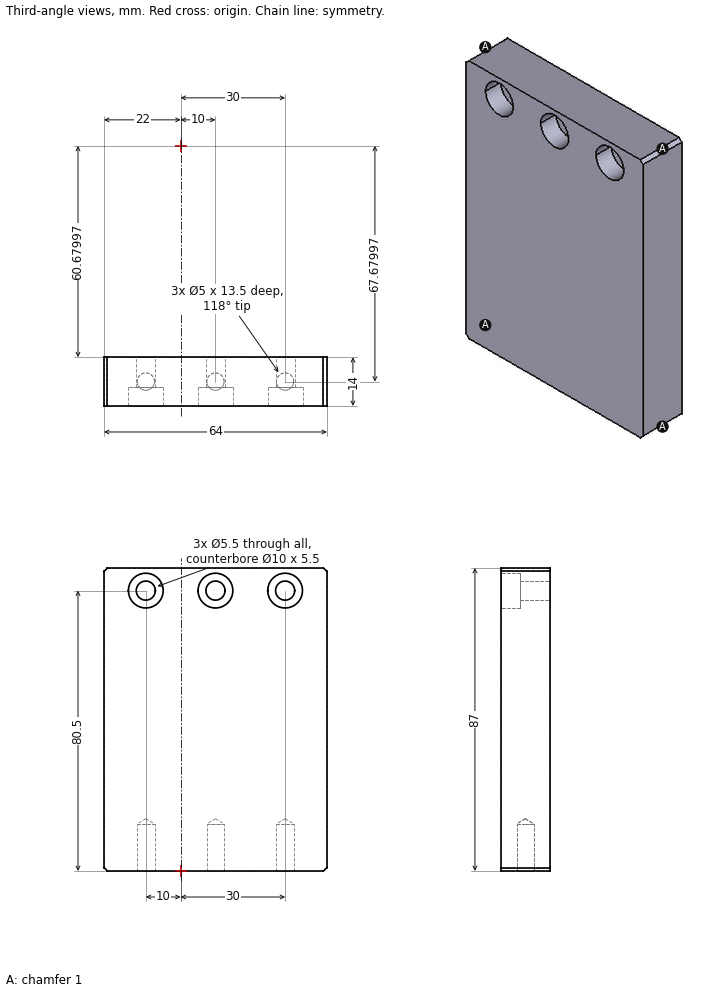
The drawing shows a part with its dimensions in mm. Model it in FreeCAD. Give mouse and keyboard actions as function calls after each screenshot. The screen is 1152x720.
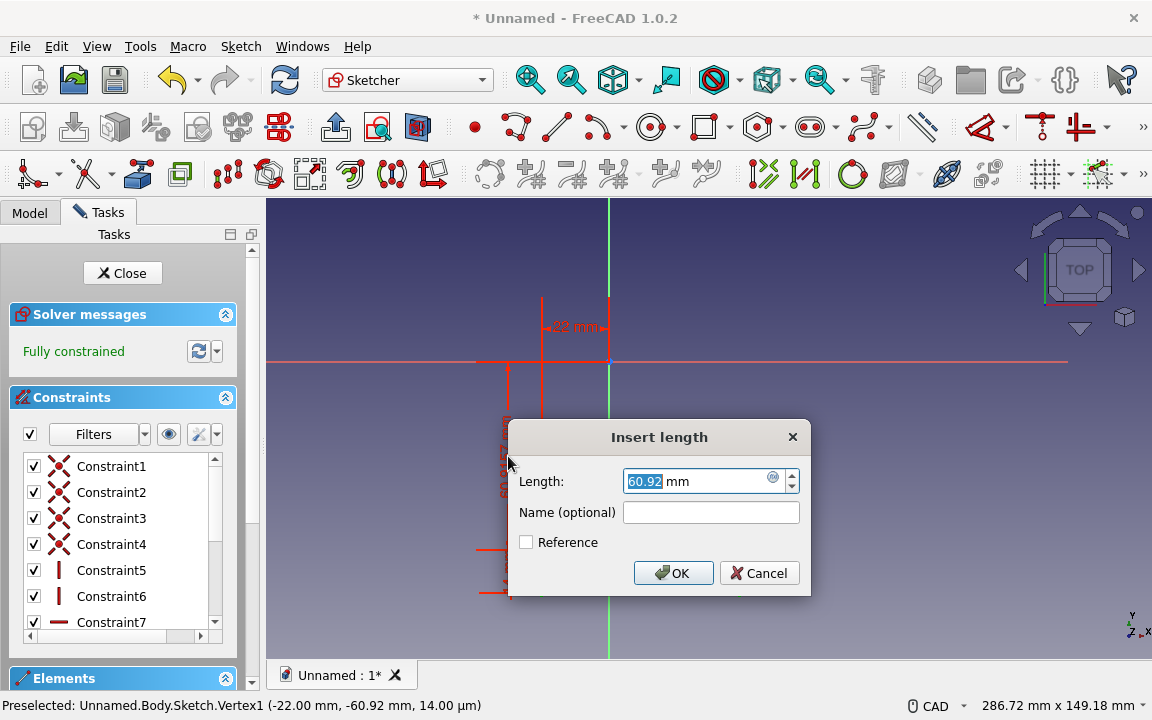
text(60.67997)
key(Return)
key(Escape)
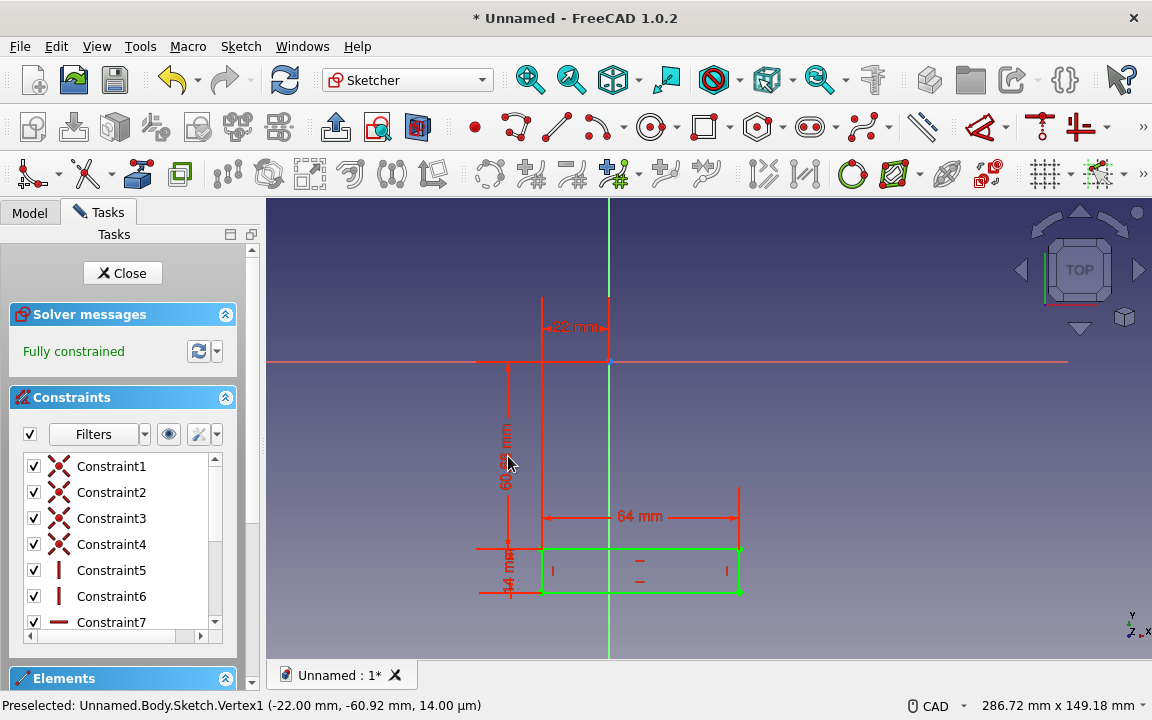
click(123, 273)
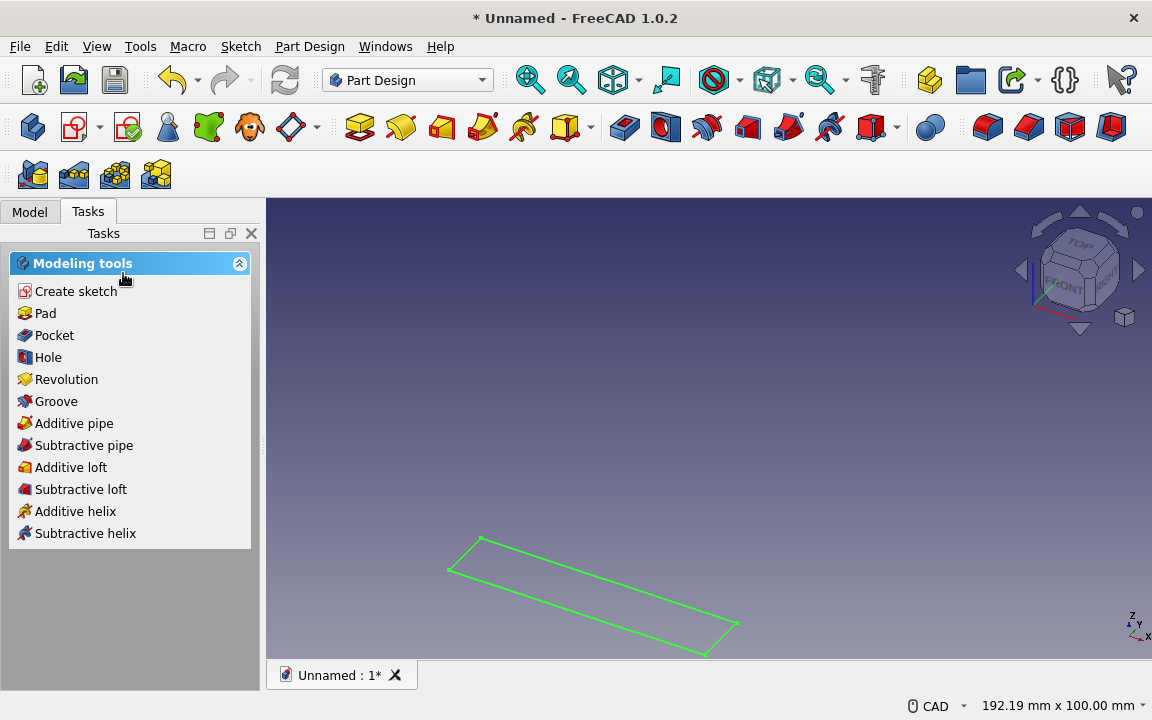
click(360, 128)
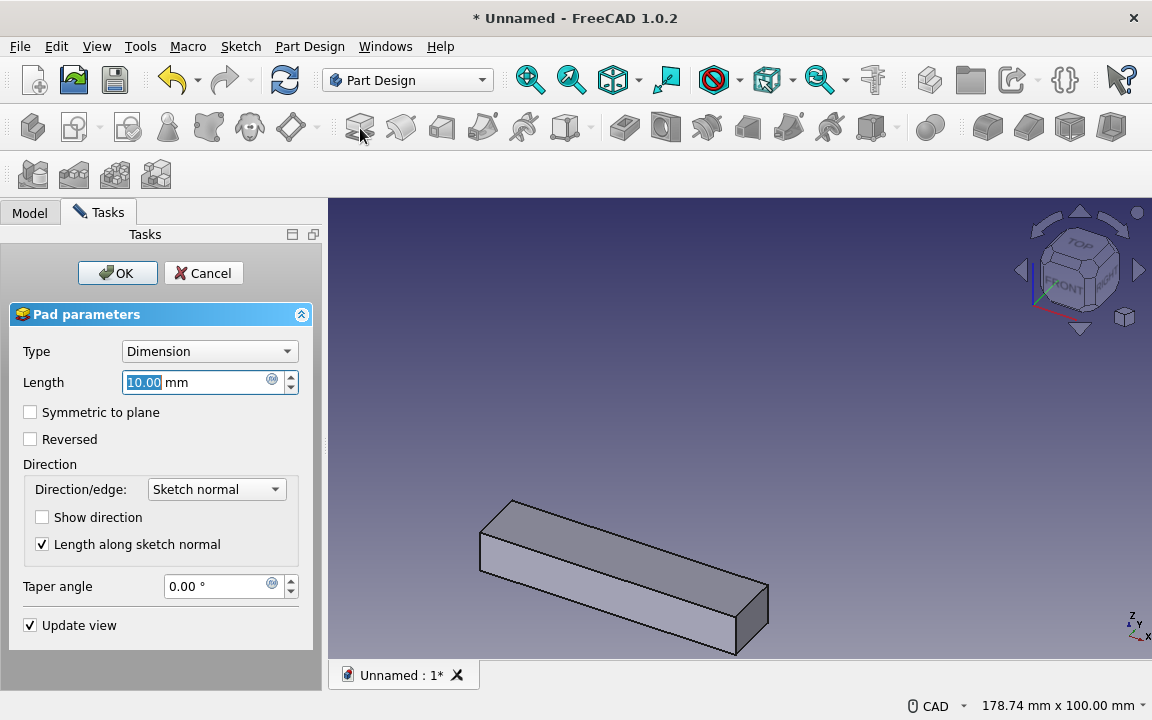
text(87)
key(Tab)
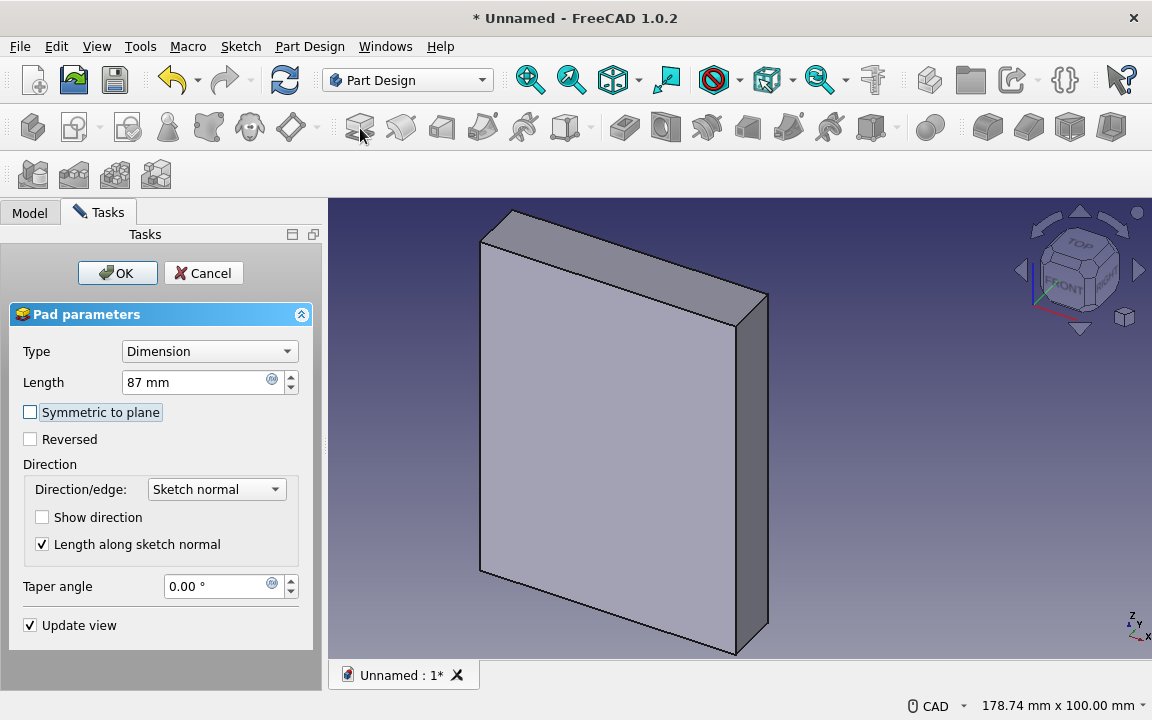
click(118, 273)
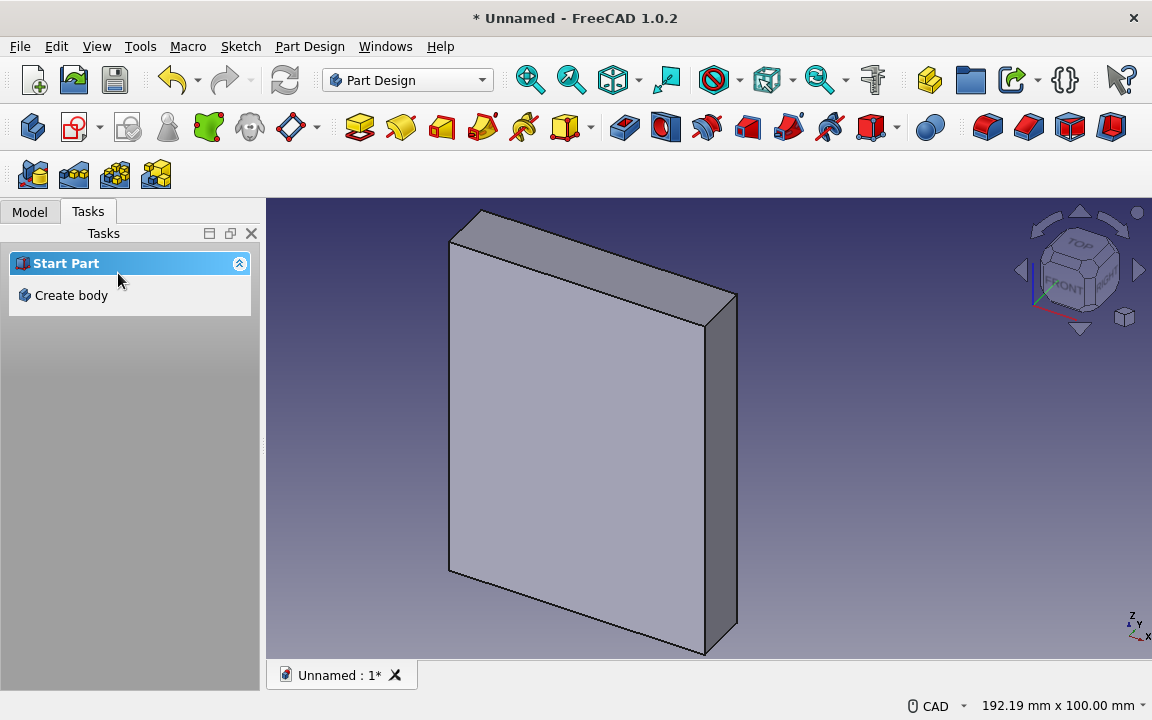
click(577, 447)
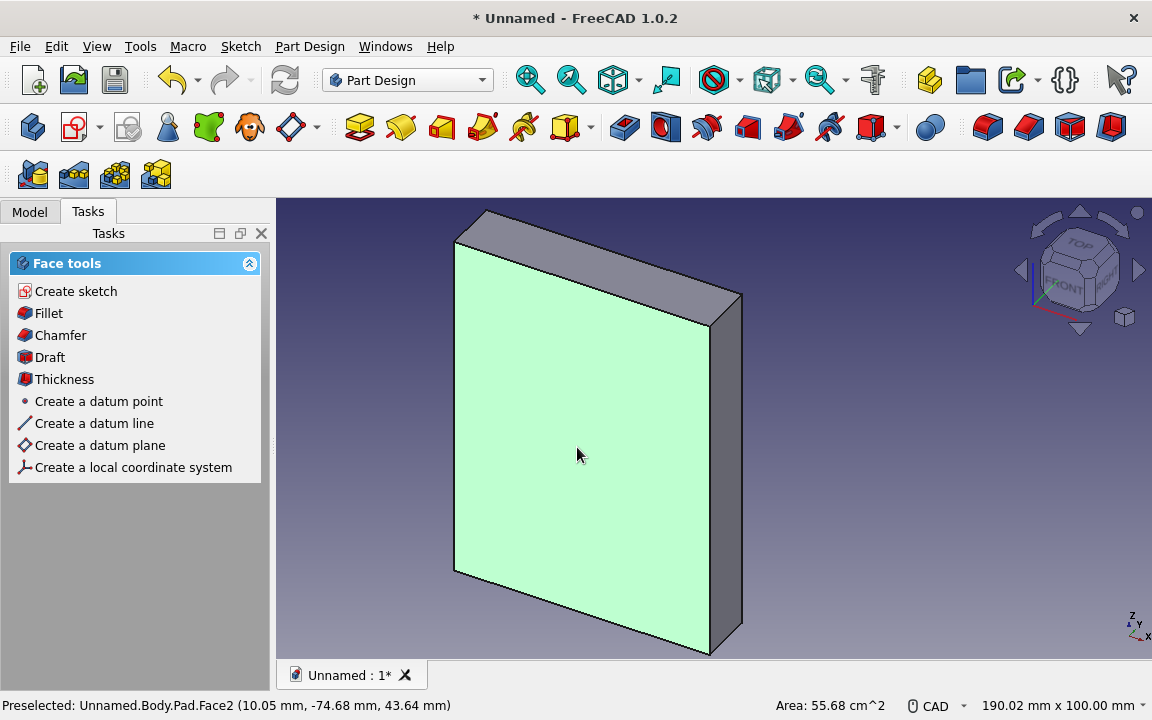
click(74, 128)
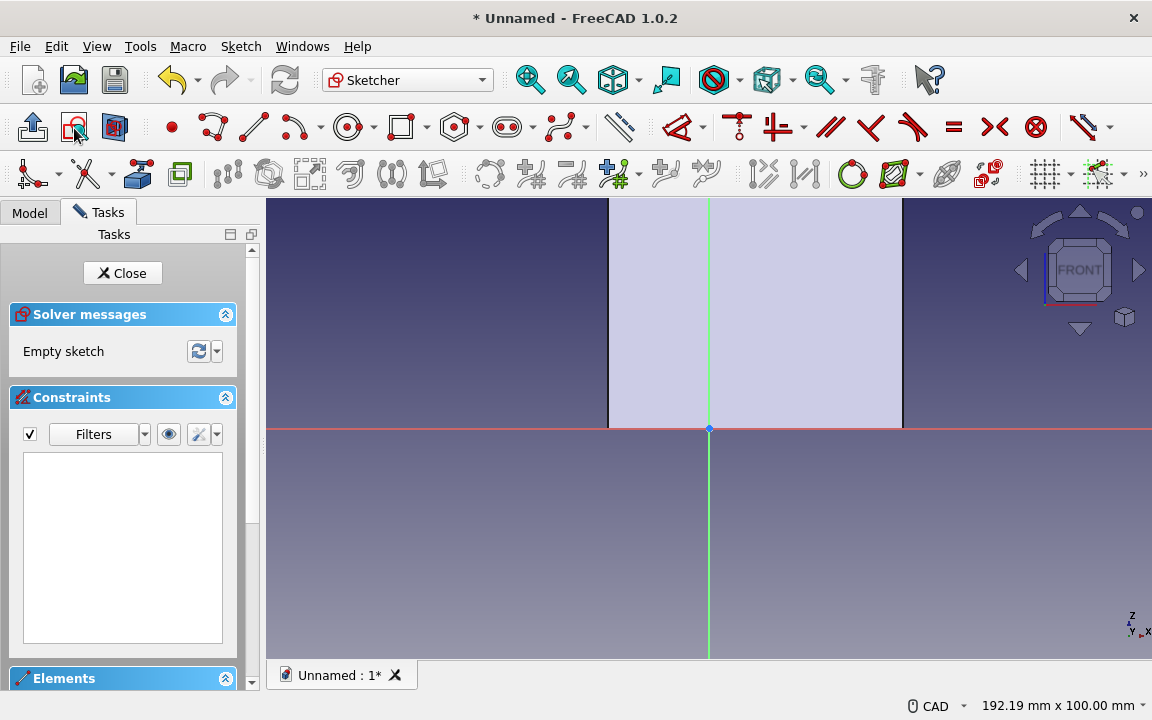
scroll(501, 631, down, 3)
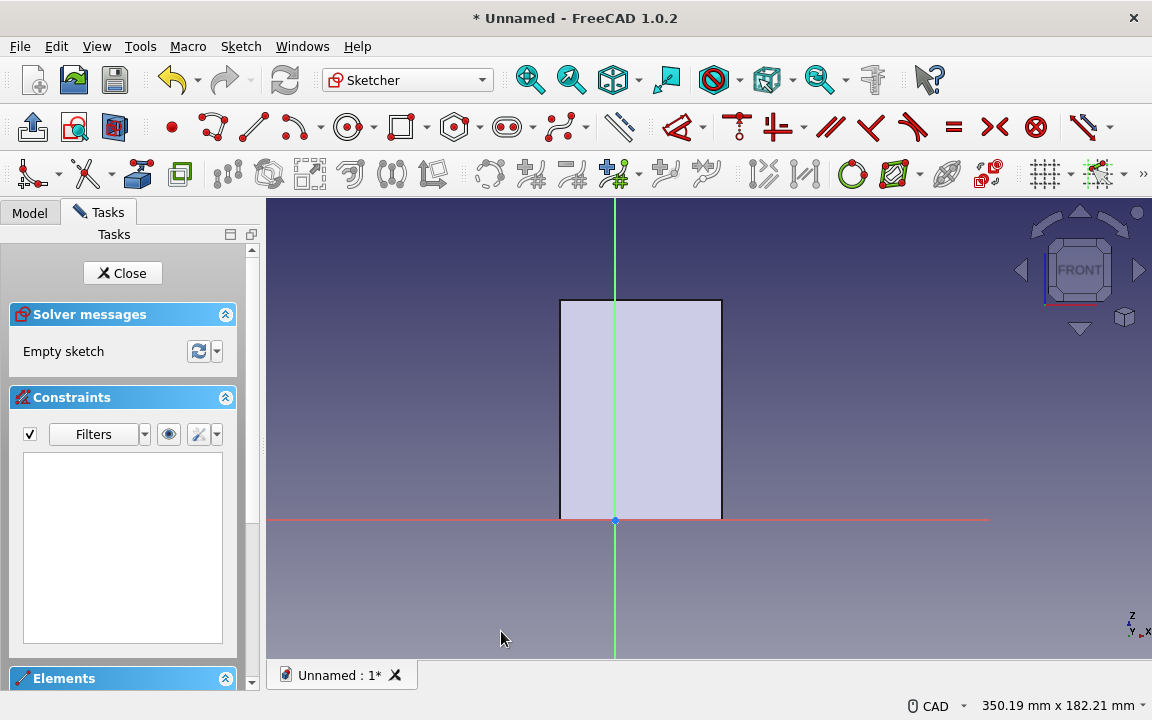
scroll(641, 387, up, 2)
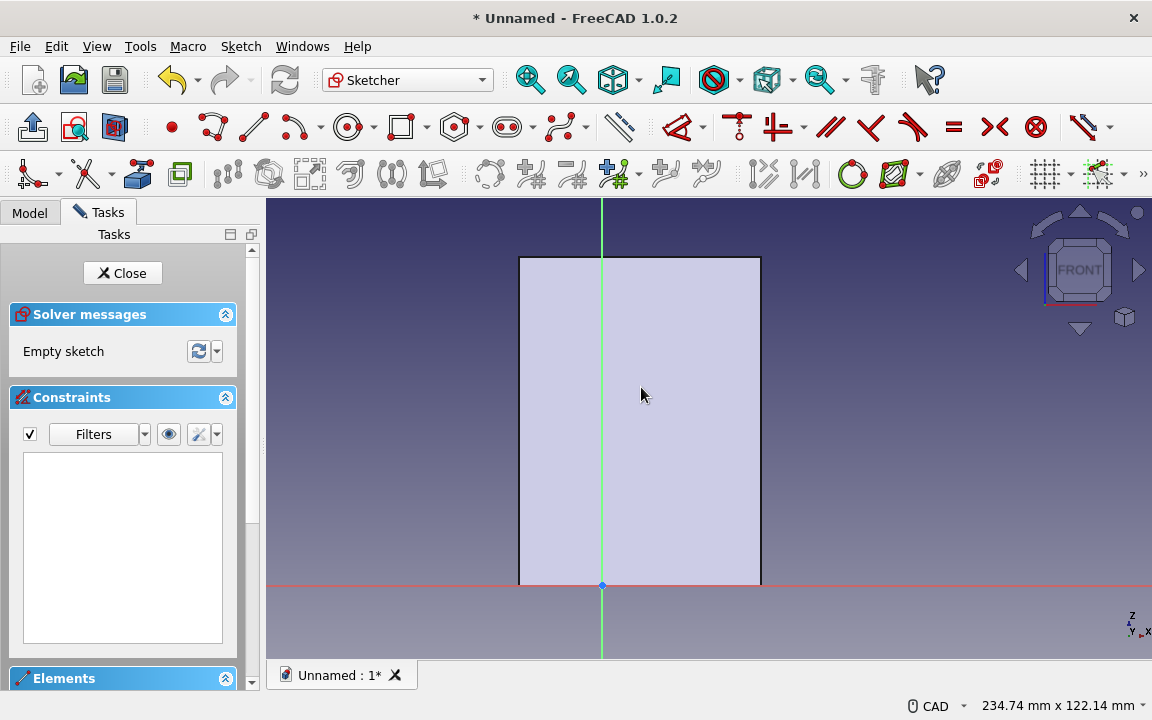
key(g)
key(c)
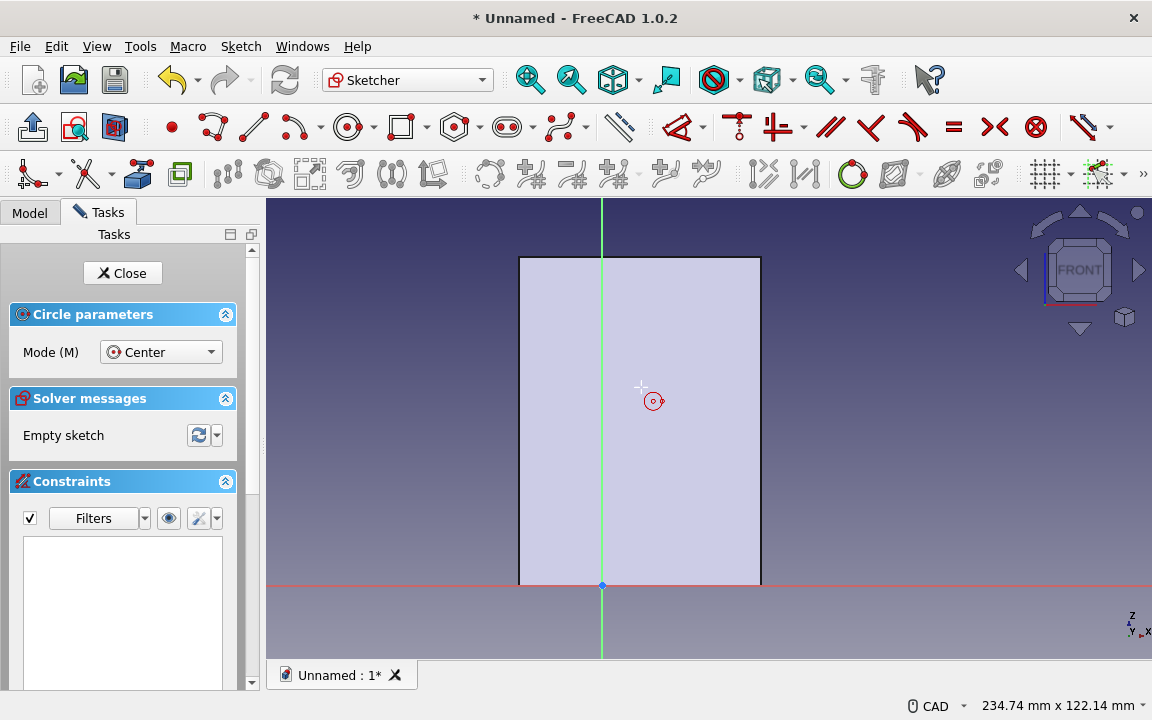
scroll(565, 282, up, 4)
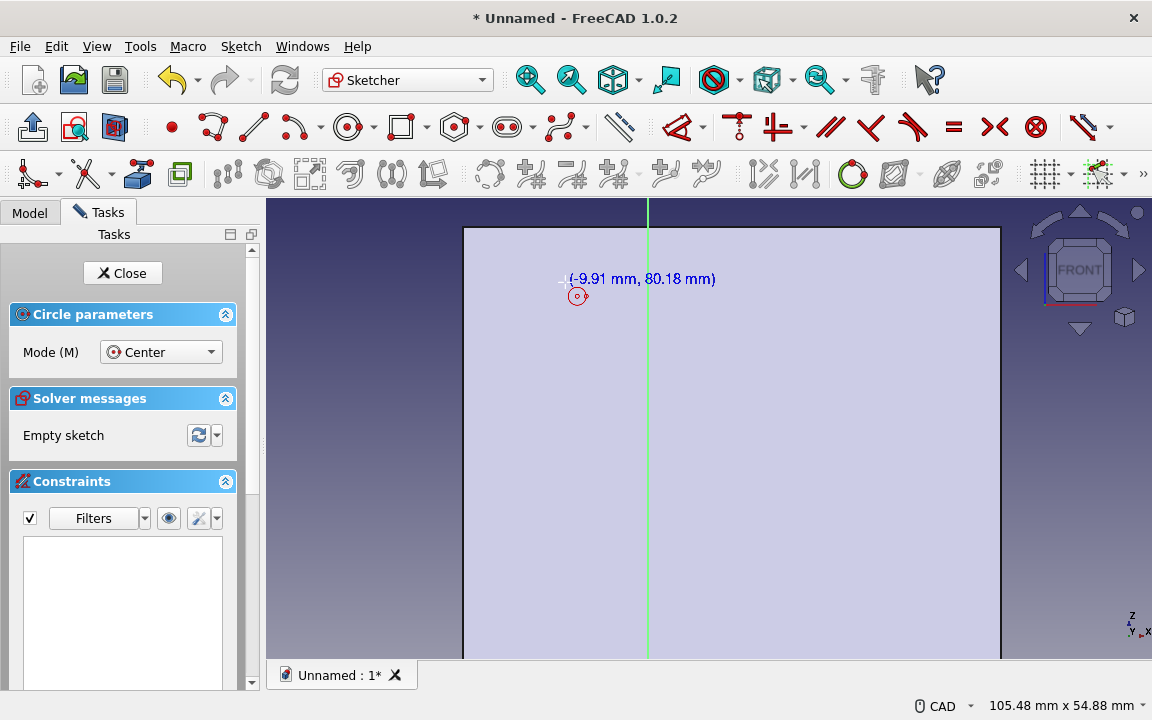
click(564, 281)
move(580, 265)